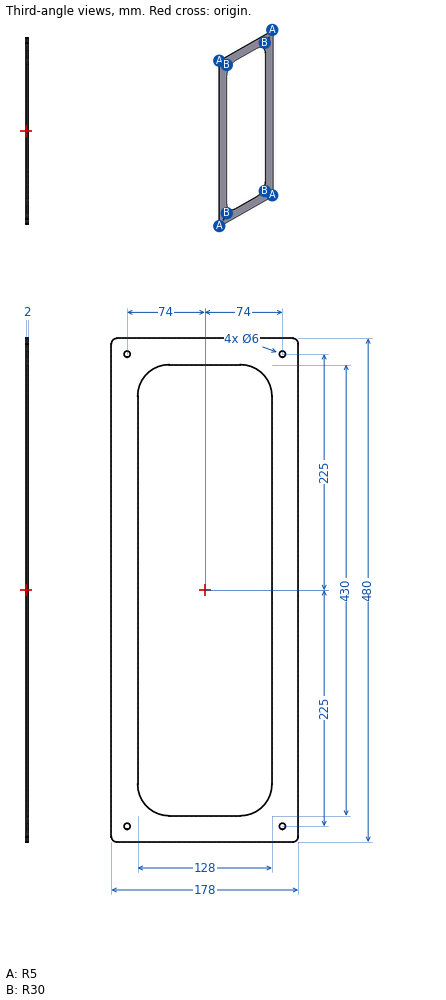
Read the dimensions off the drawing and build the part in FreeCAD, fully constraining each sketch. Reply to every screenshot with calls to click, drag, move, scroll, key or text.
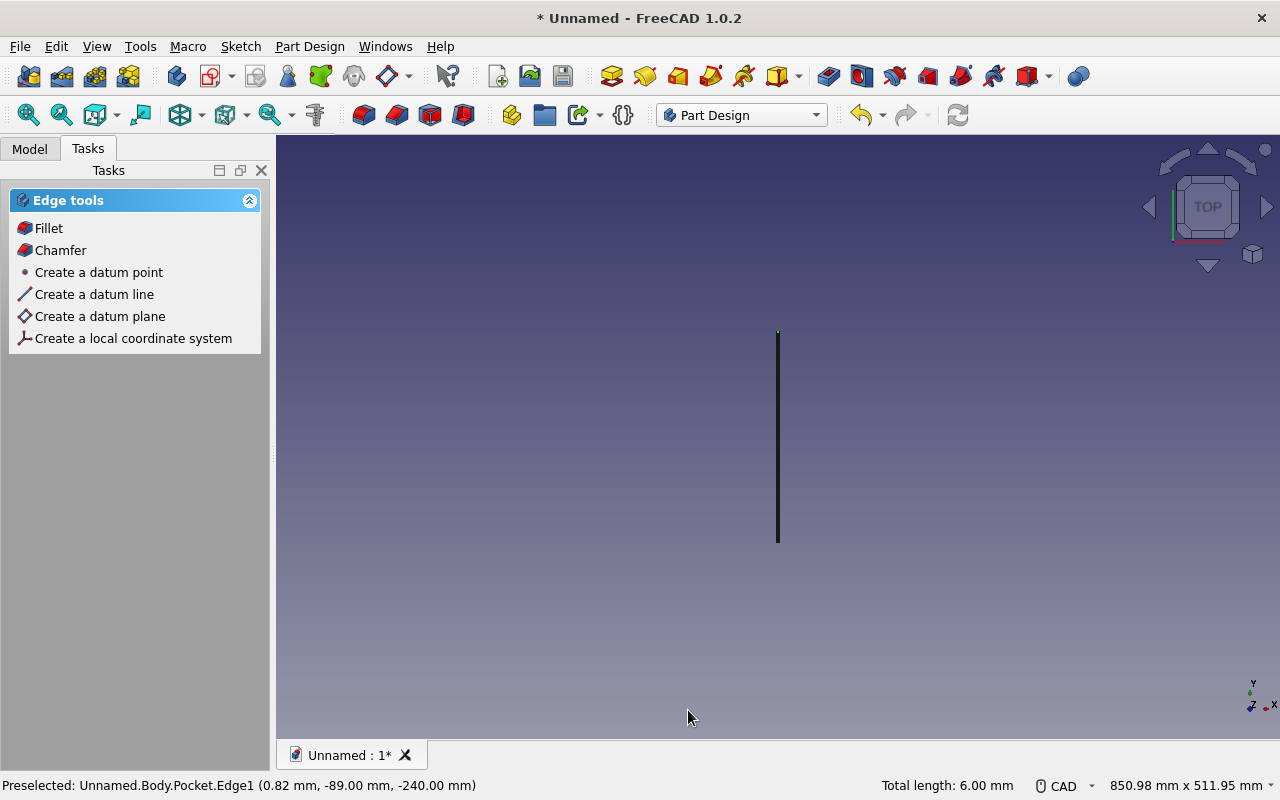
key(v)
key(f)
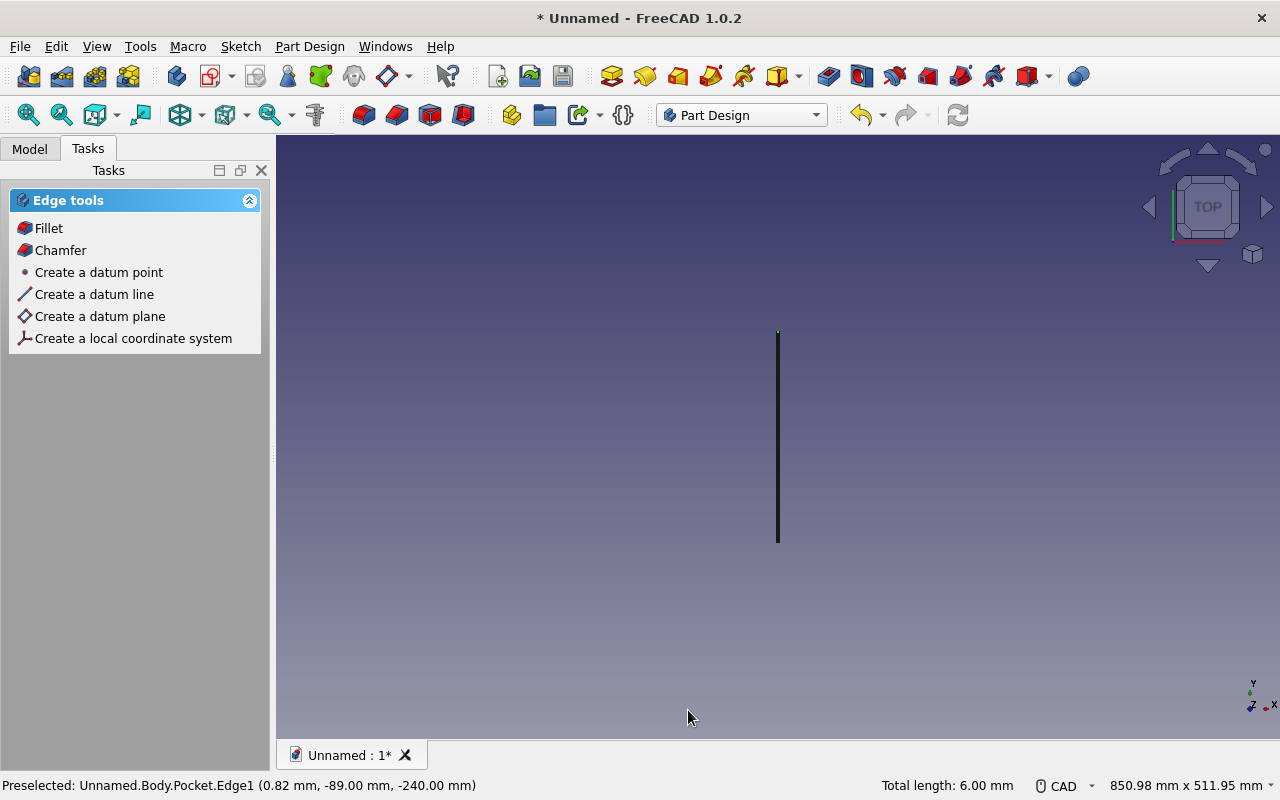
scroll(778, 541, up, 15)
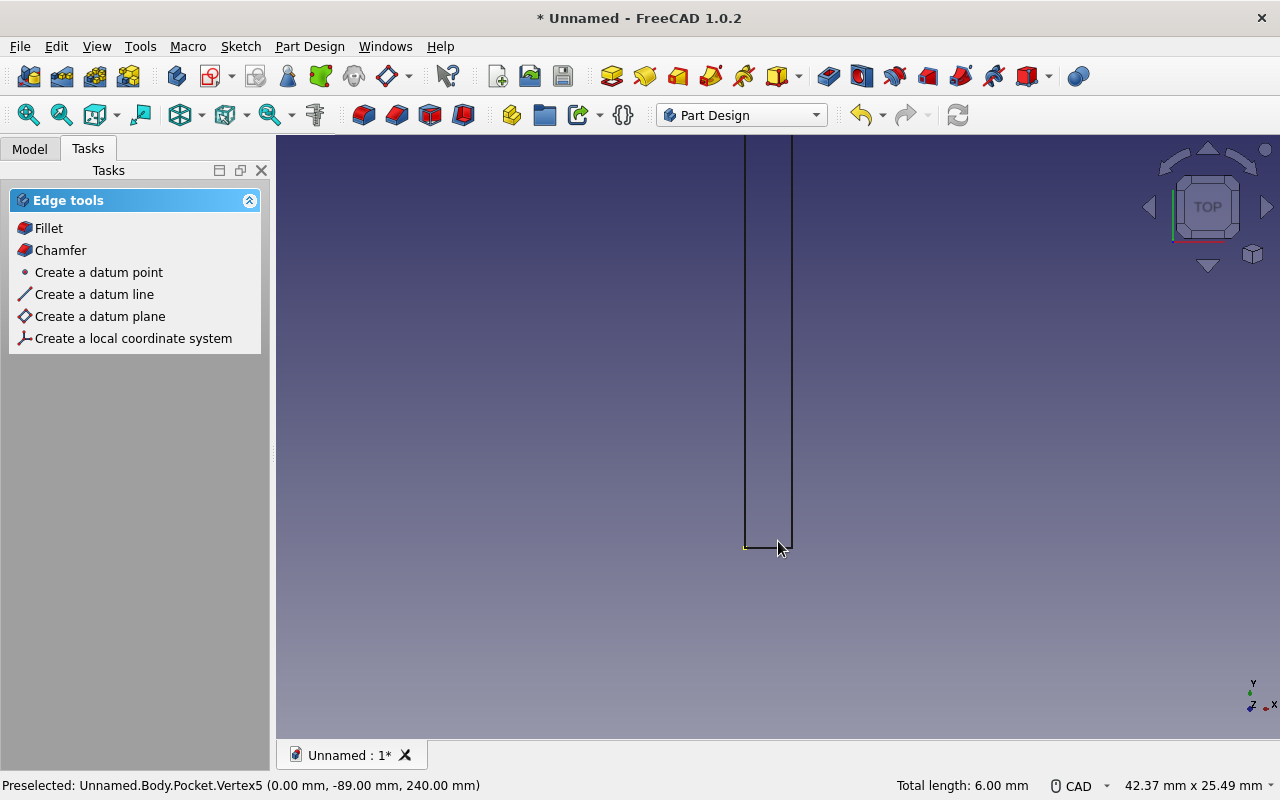
click(768, 547, ctrl)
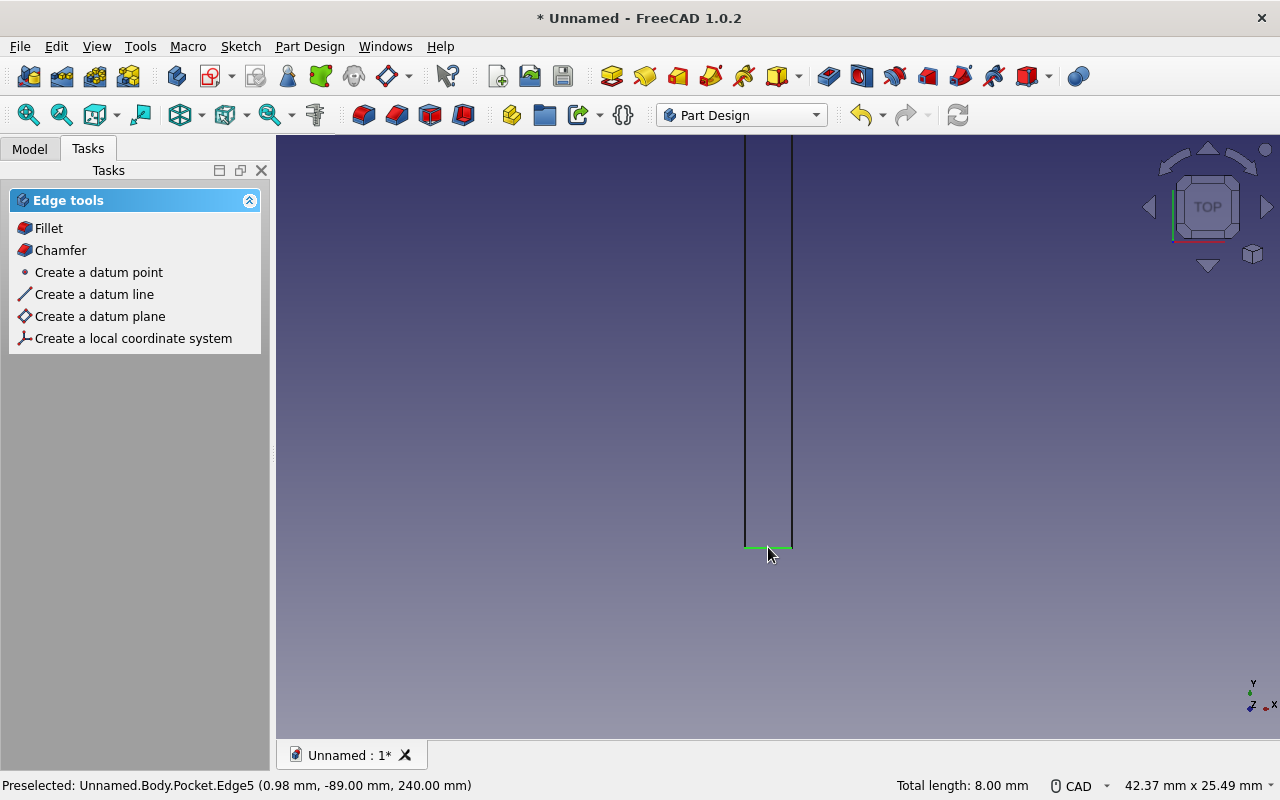
key(v)
key(1)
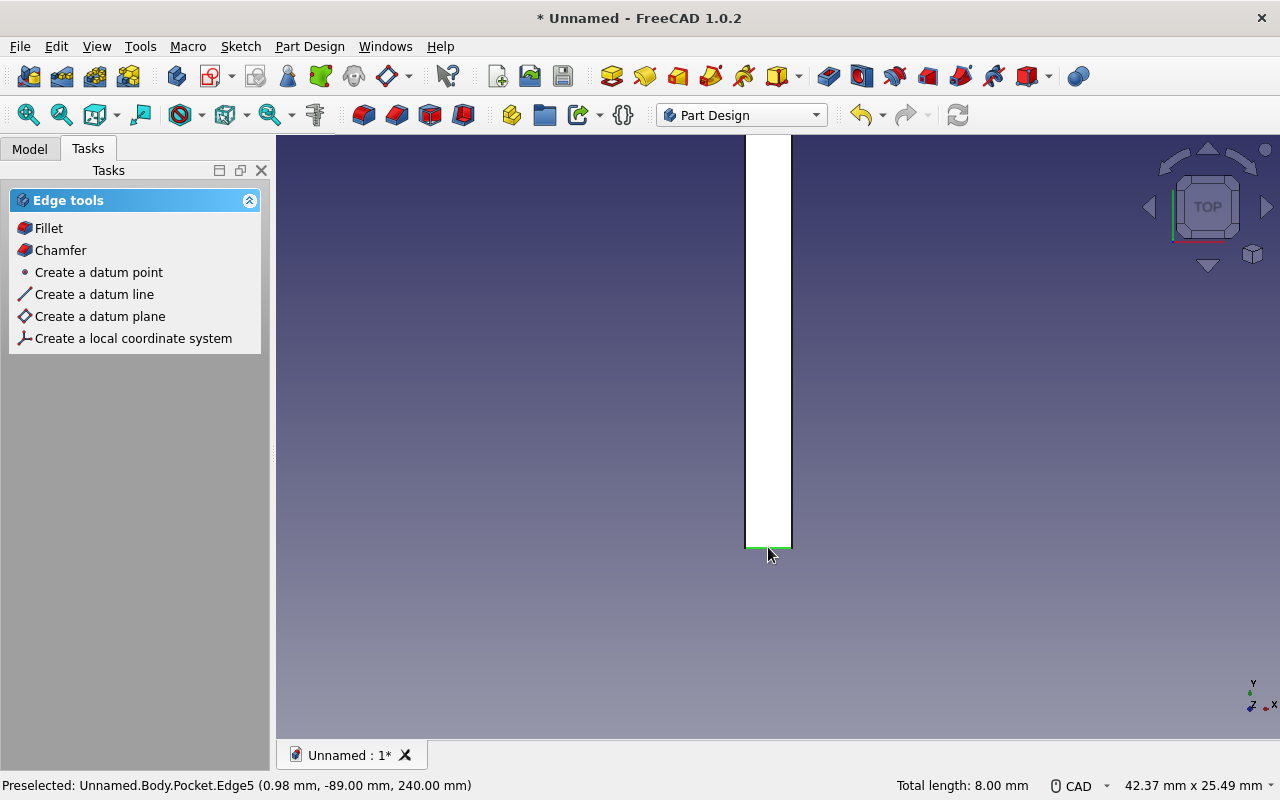
click(364, 116)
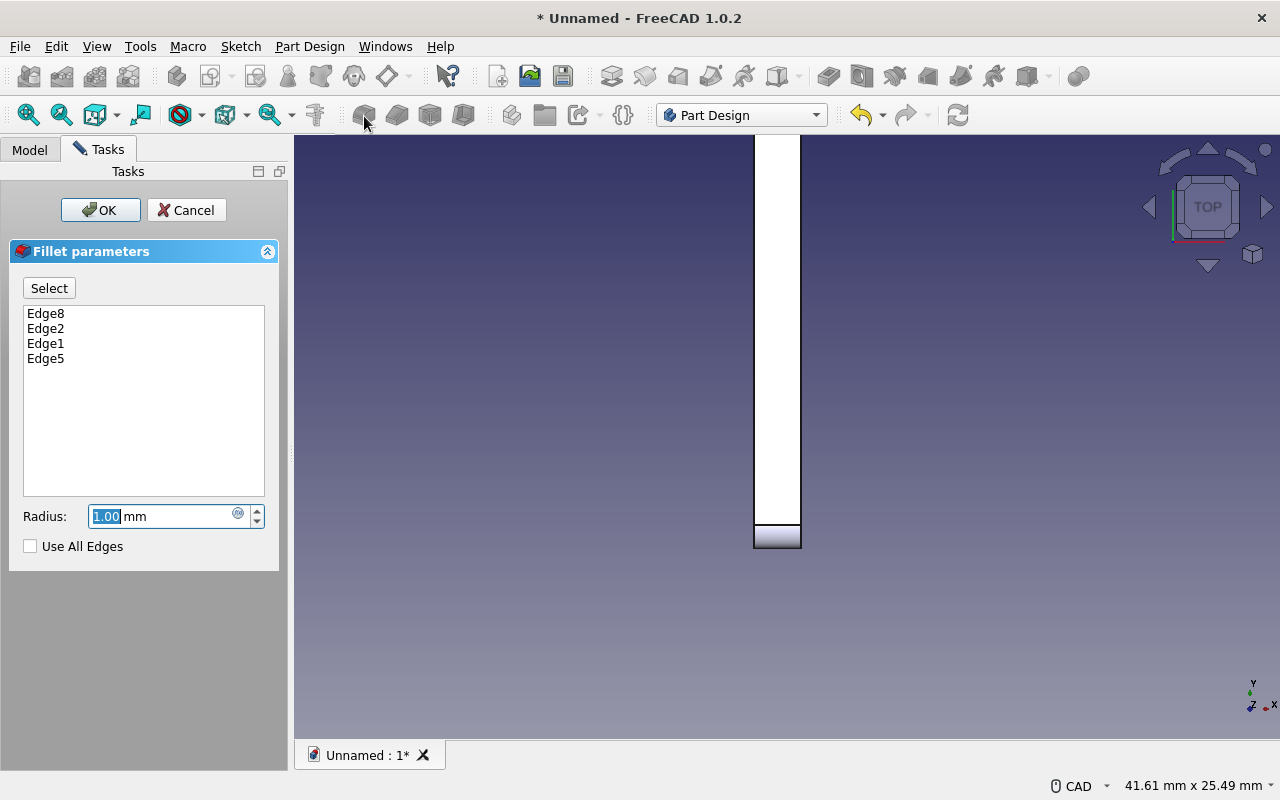
text(5)
key(Tab)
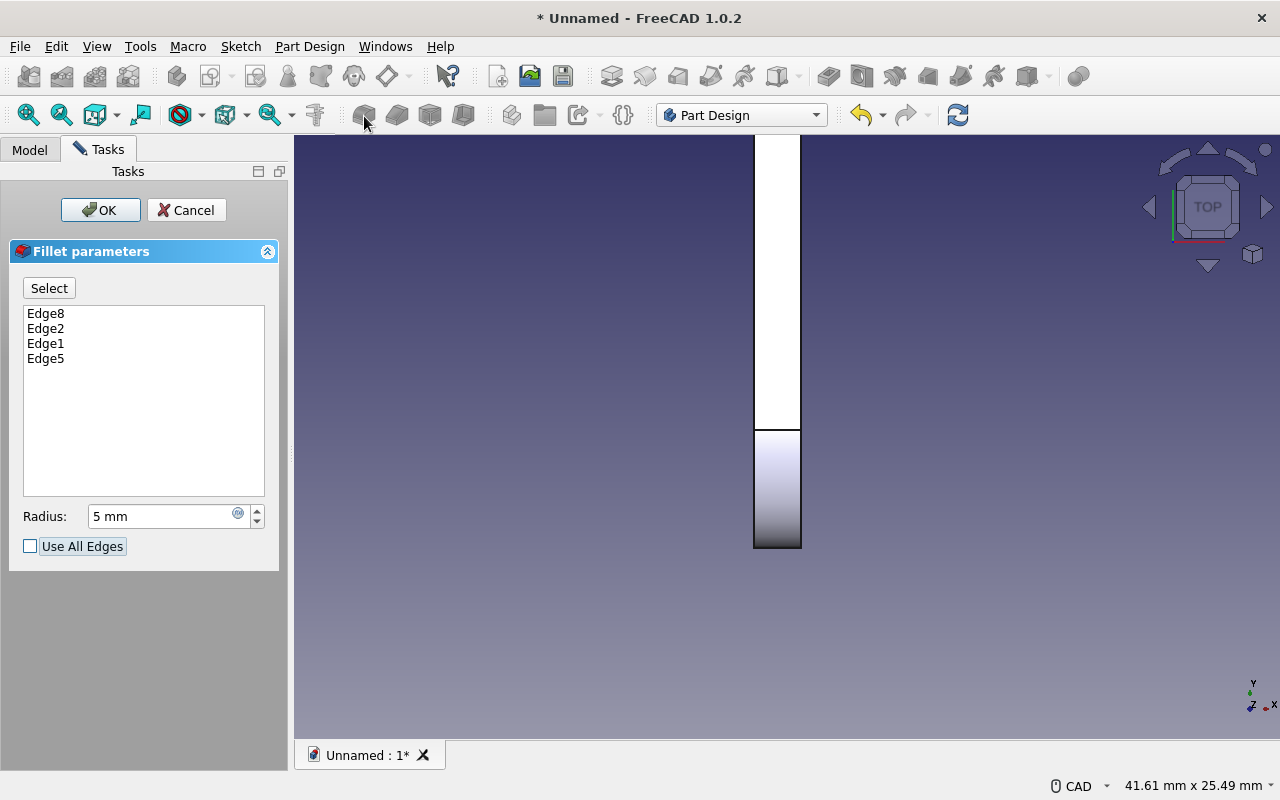
click(101, 210)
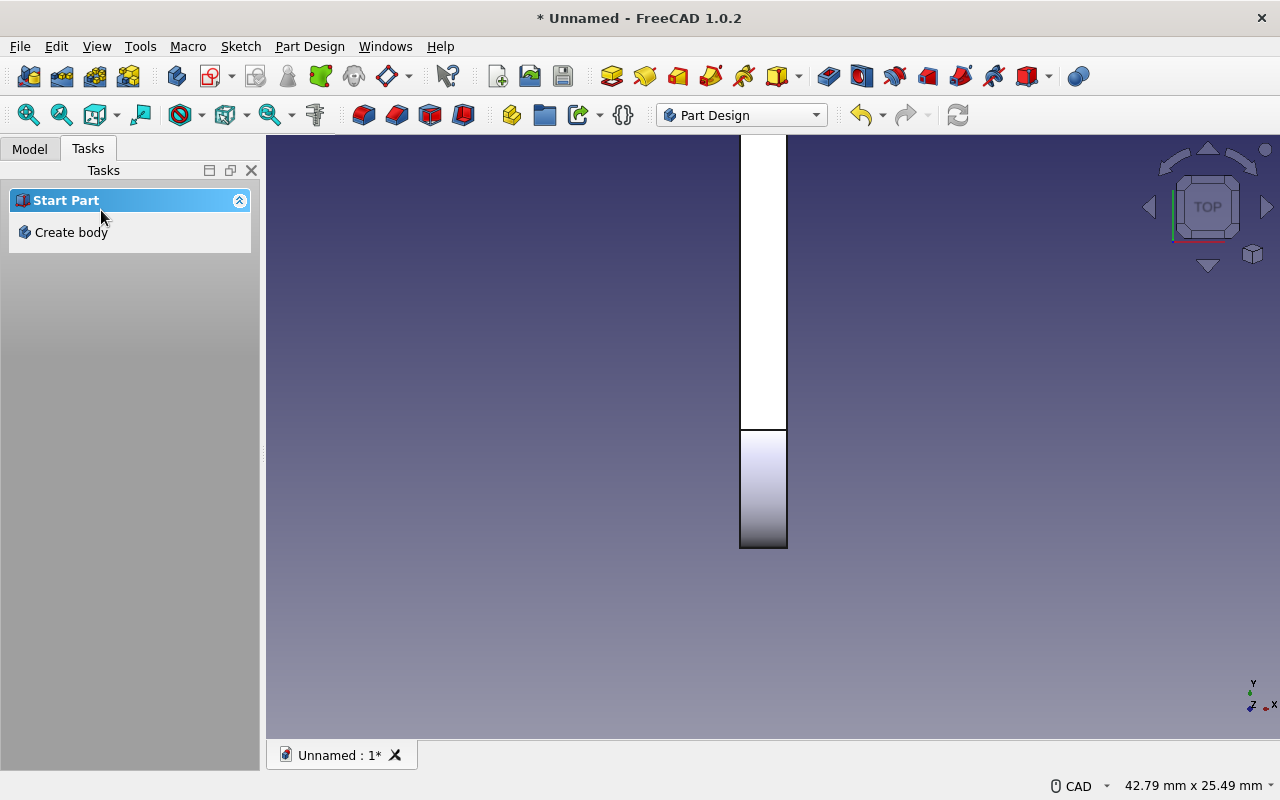
key(v)
key(f)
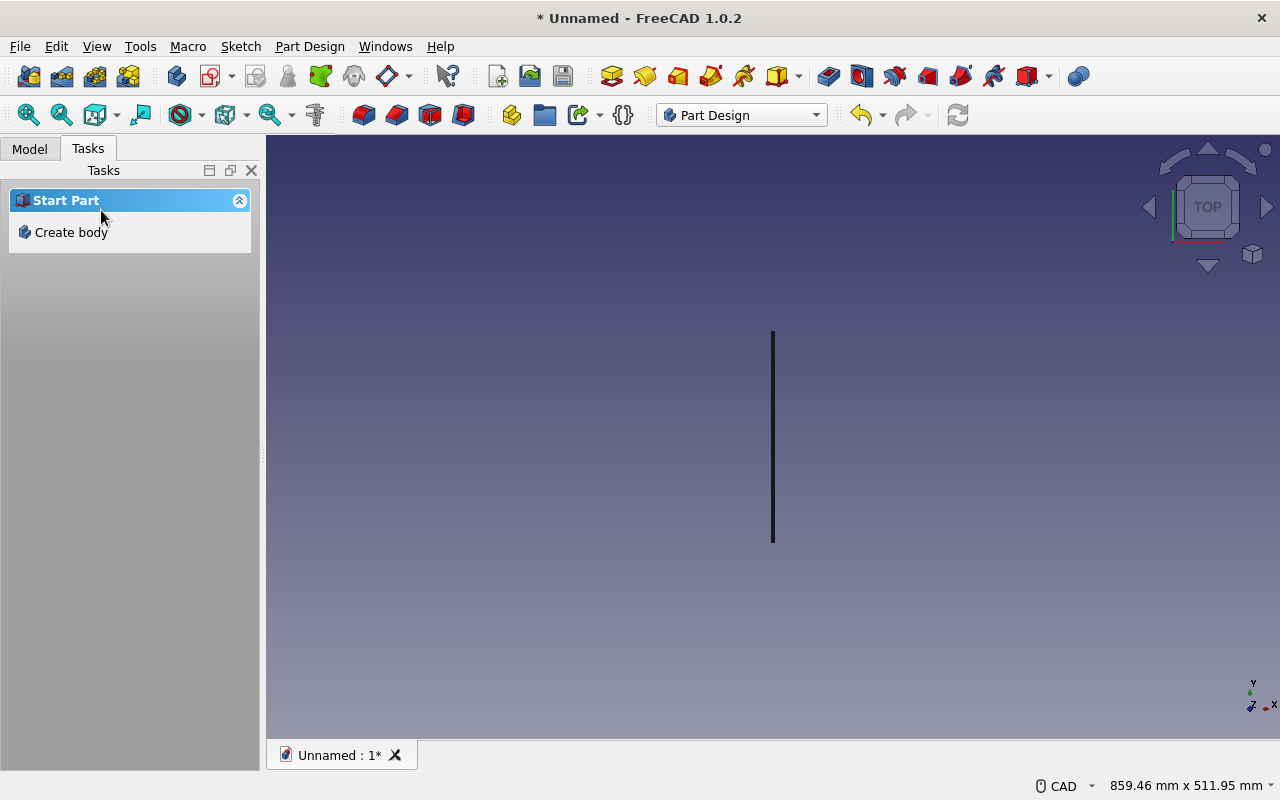
key(0)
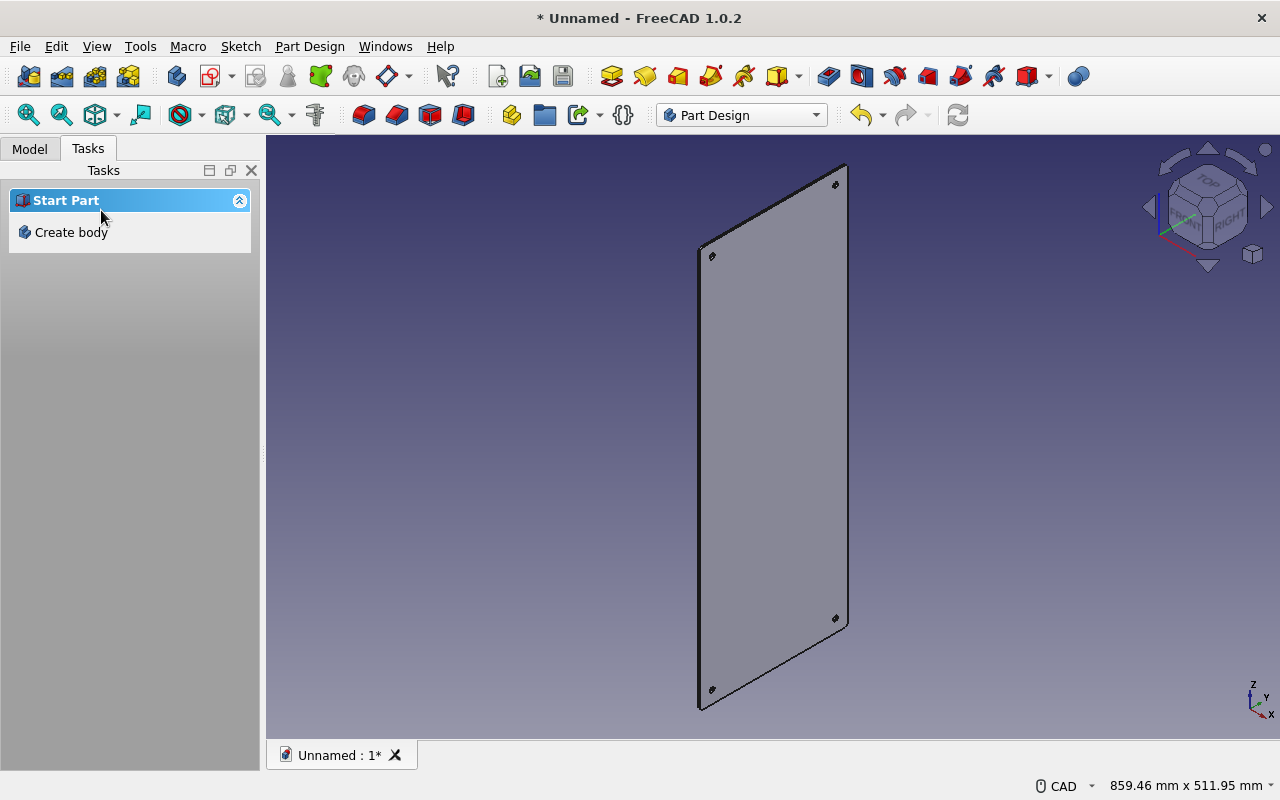
click(774, 569)